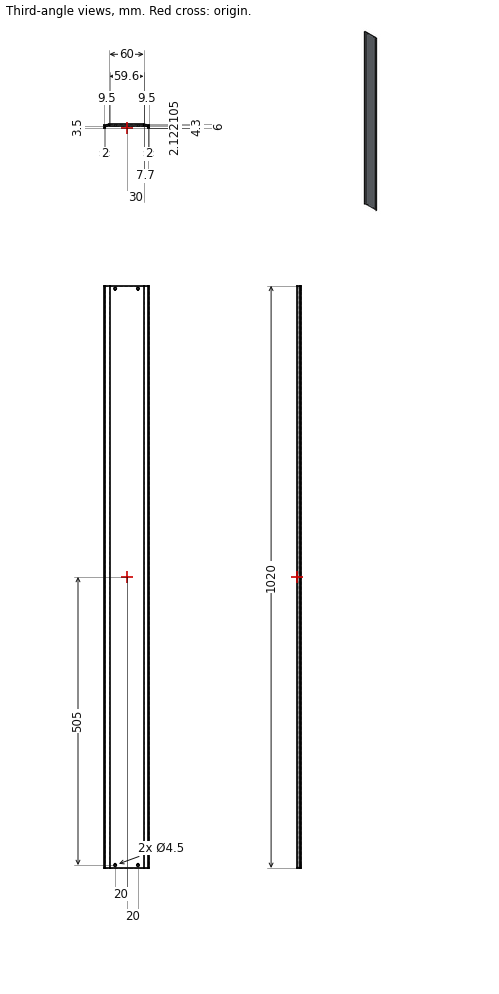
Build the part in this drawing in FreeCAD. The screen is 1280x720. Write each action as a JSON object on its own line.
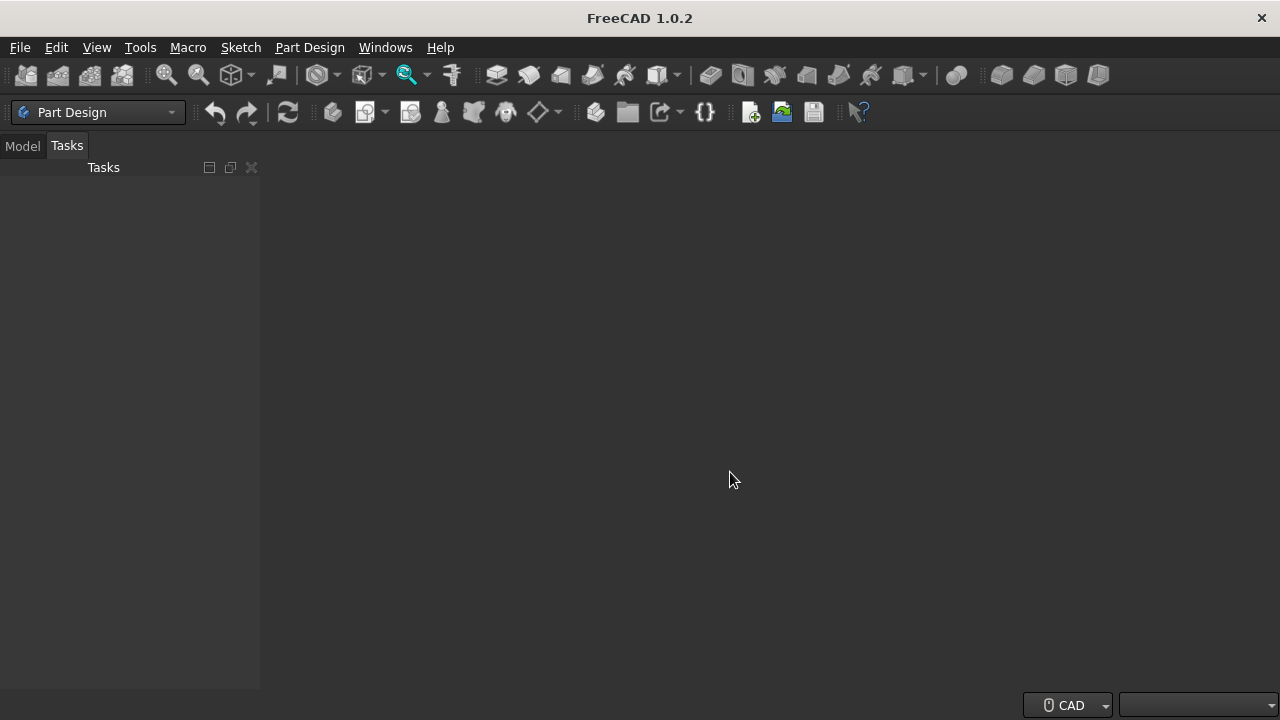
{"action": "key", "text": "ctrl+n"}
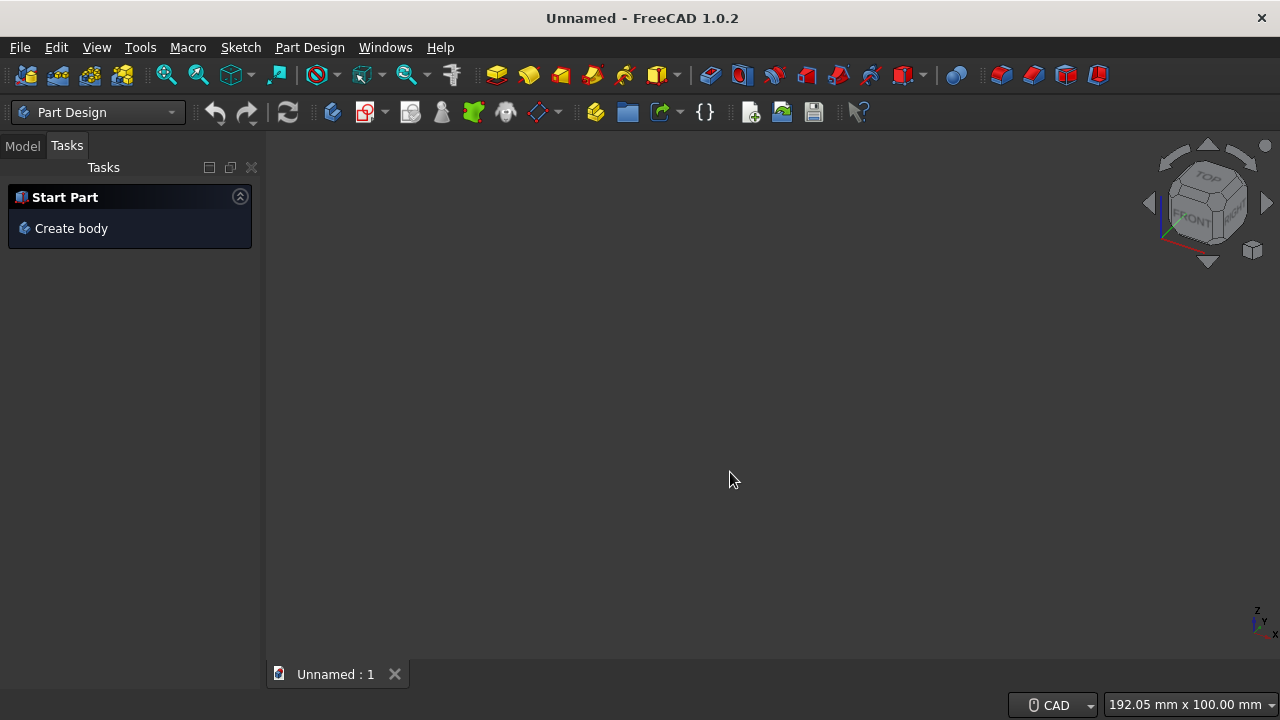
{"action": "left_click", "coordinate": [366, 112]}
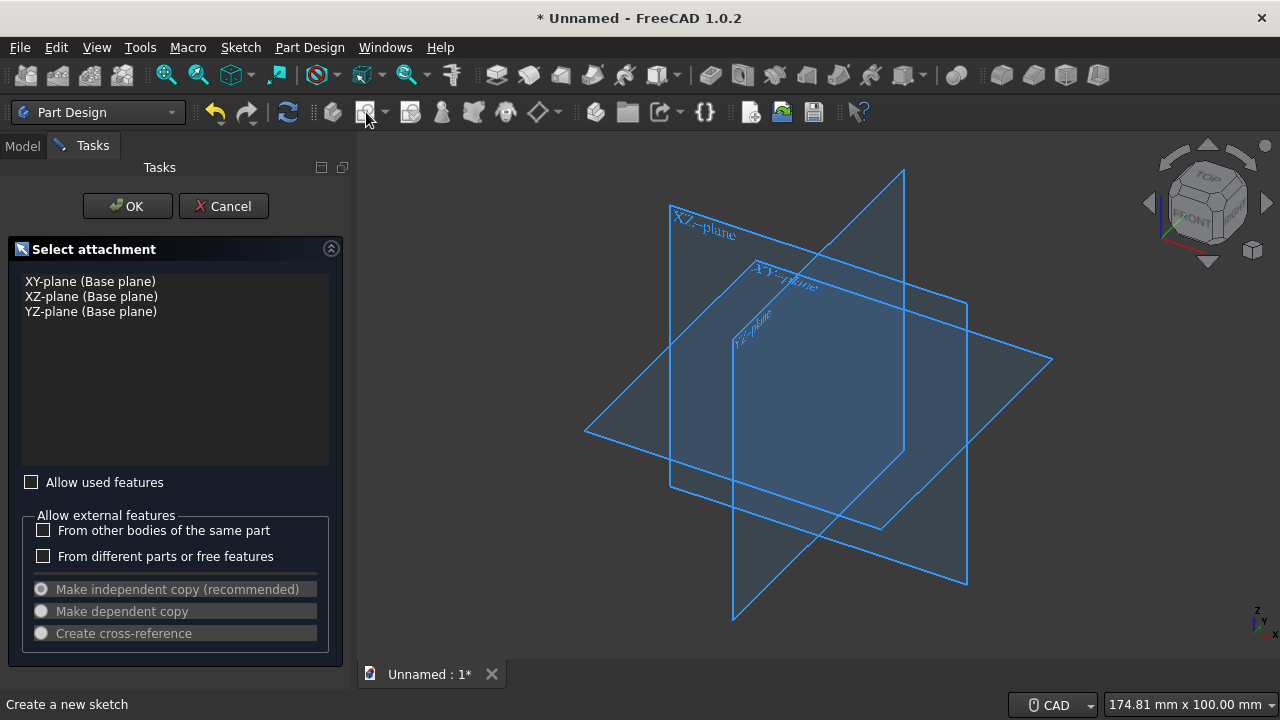
{"action": "left_click", "coordinate": [82, 282]}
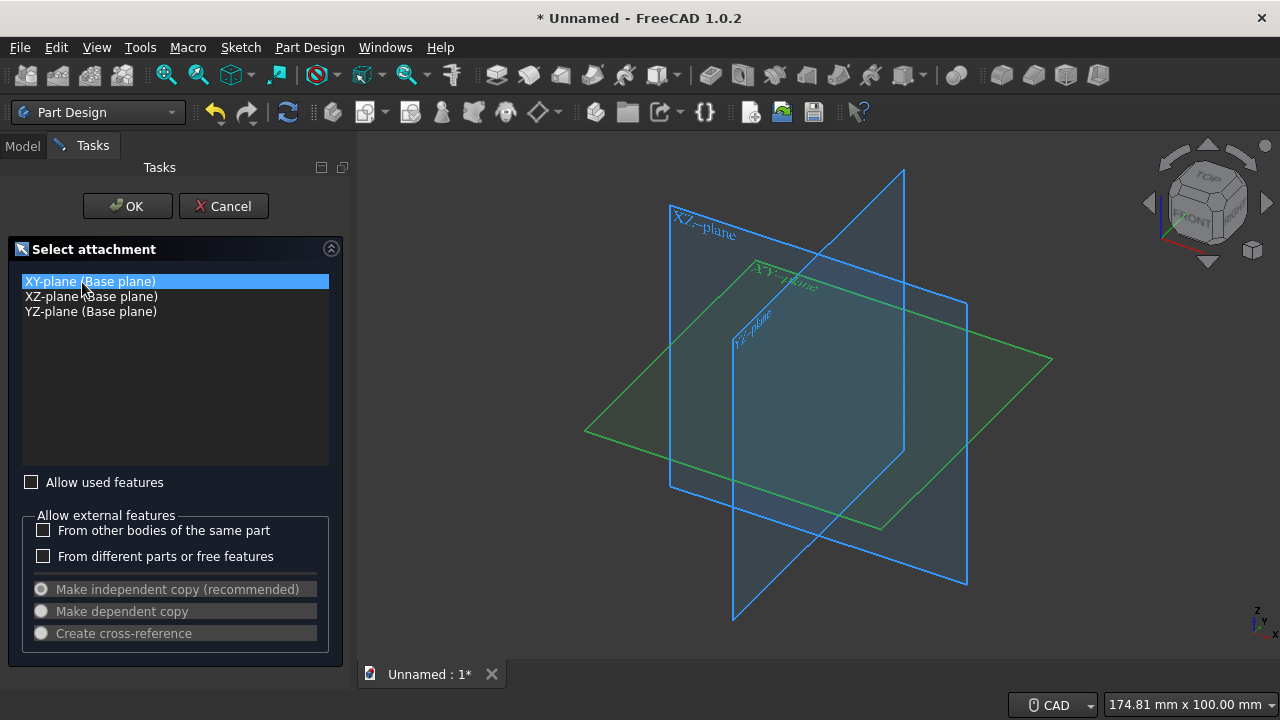
{"action": "left_click", "coordinate": [128, 206]}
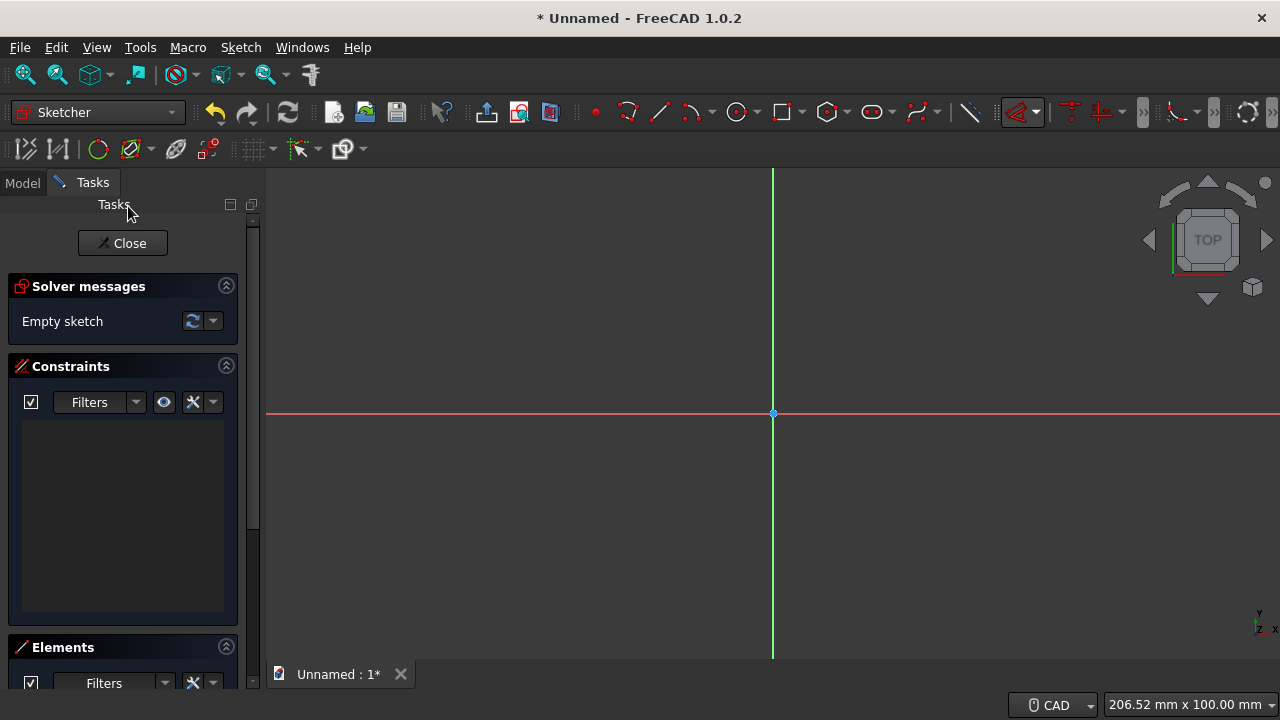
{"action": "scroll", "coordinate": [912, 369], "scroll_direction": "up", "scroll_amount": 2}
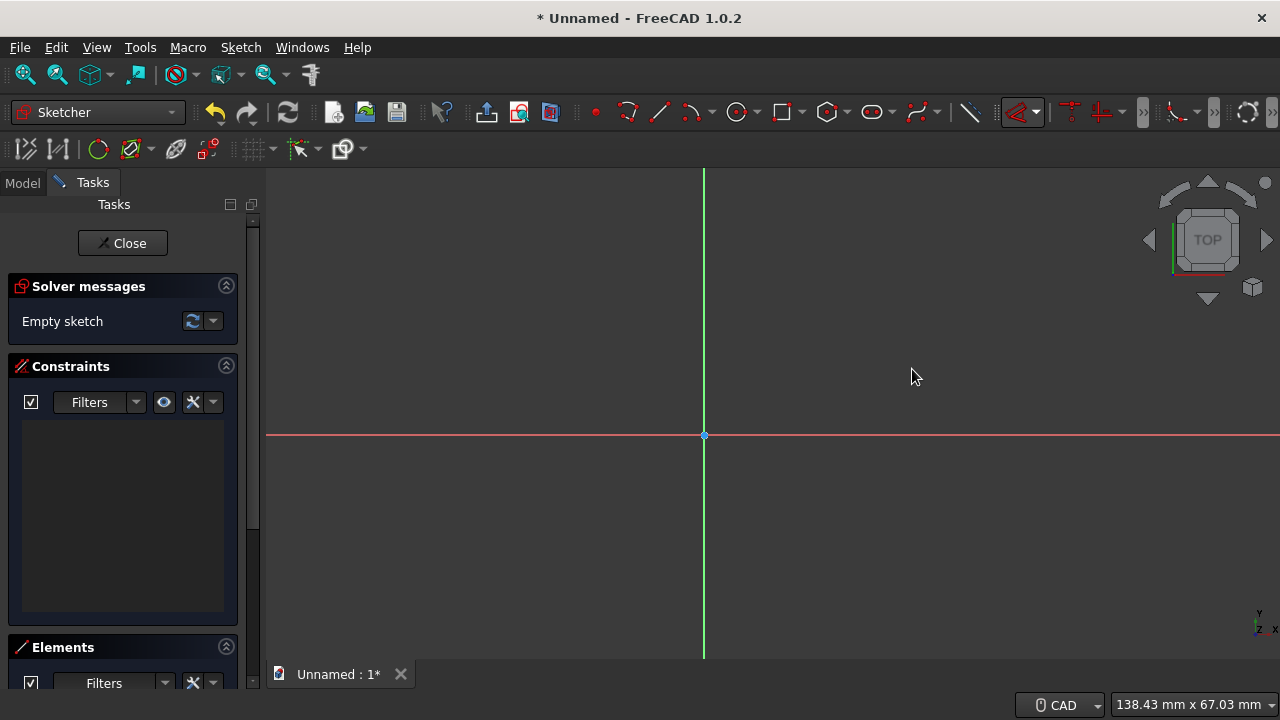
{"action": "key", "text": "g m"}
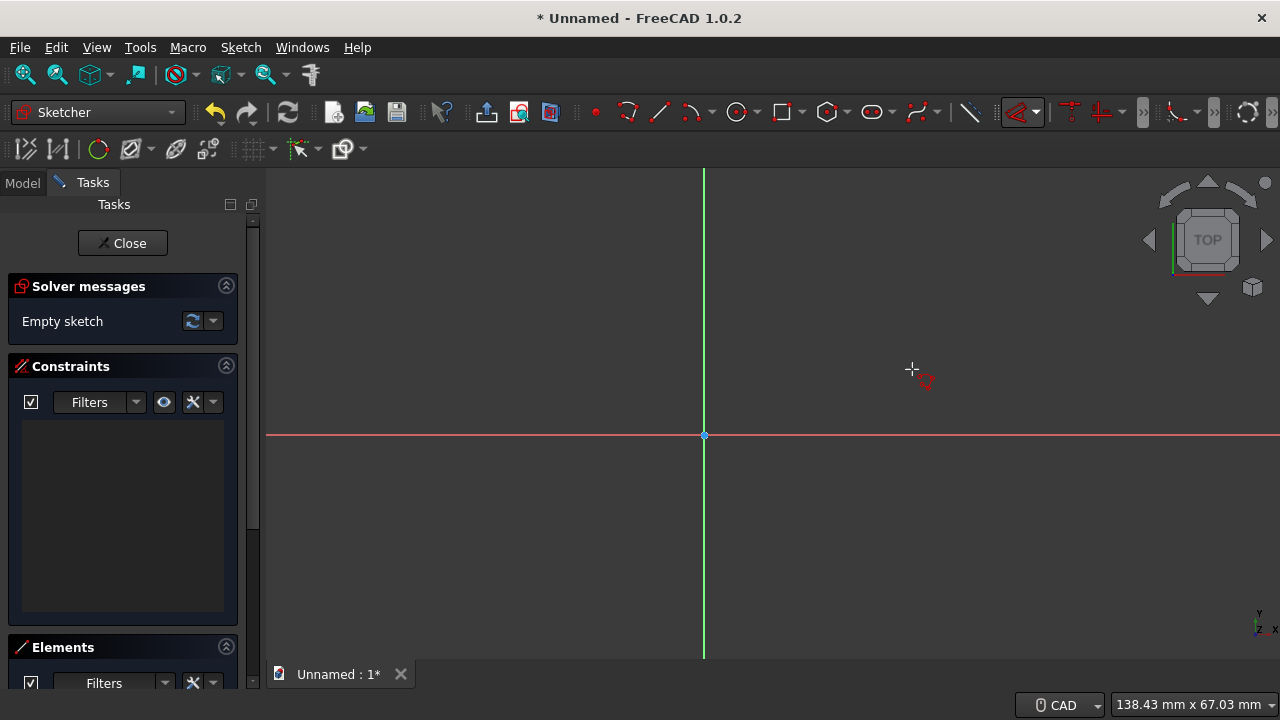
{"action": "left_click", "coordinate": [486, 410]}
{"action": "left_click", "coordinate": [923, 410]}
{"action": "left_click", "coordinate": [979, 420]}
{"action": "left_click", "coordinate": [979, 435]}
{"action": "left_click", "coordinate": [994, 426]}
{"action": "left_click", "coordinate": [994, 404]}
{"action": "left_click", "coordinate": [924, 391]}
{"action": "left_click", "coordinate": [485, 391]}
{"action": "left_click", "coordinate": [415, 404]}
{"action": "left_click", "coordinate": [415, 435]}
{"action": "left_click", "coordinate": [430, 426]}
{"action": "left_click", "coordinate": [430, 420]}
{"action": "left_click", "coordinate": [486, 411]}
{"action": "key", "text": "Escape"}
{"action": "key", "text": "Escape"}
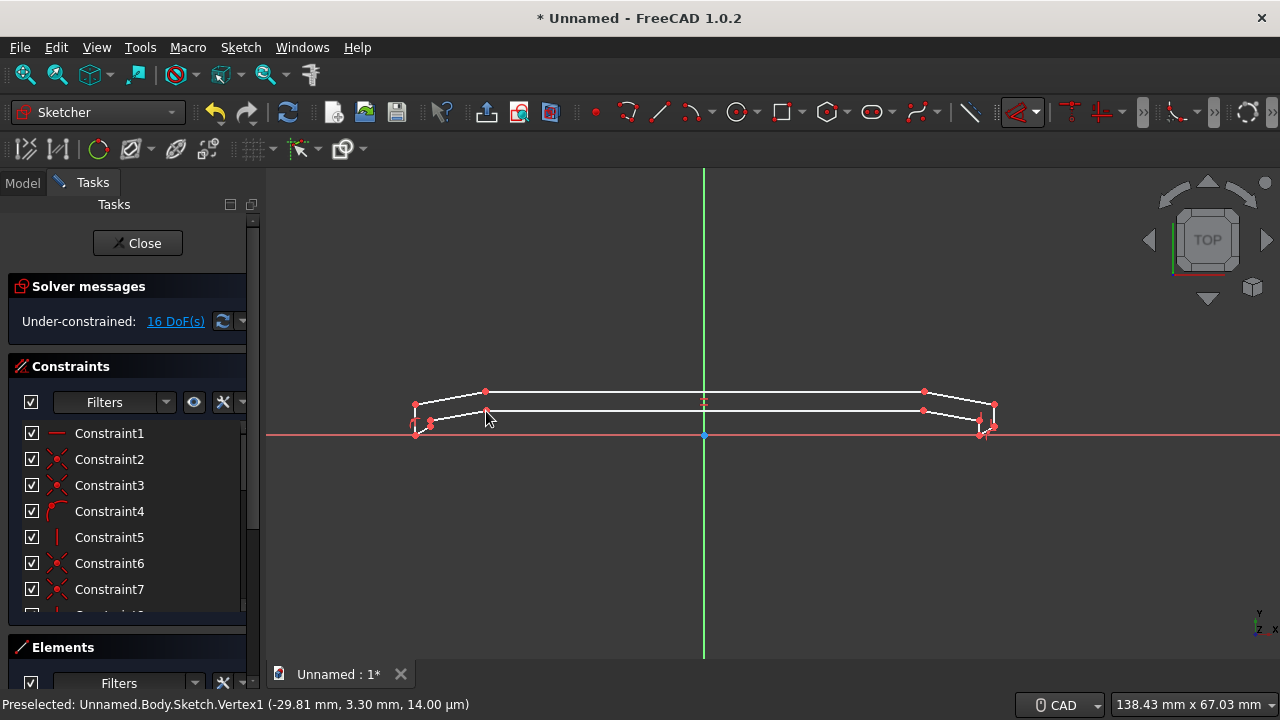
{"action": "scroll", "coordinate": [985, 432], "scroll_direction": "up", "scroll_amount": 5}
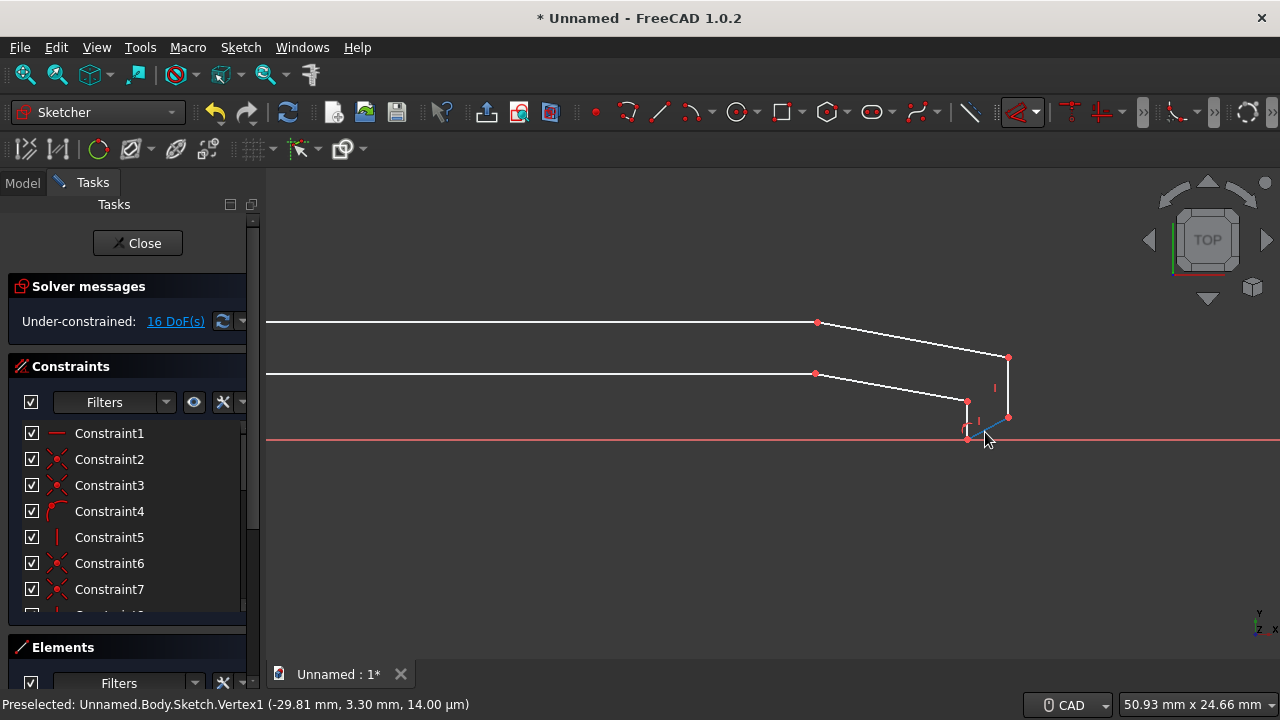
{"action": "left_click", "coordinate": [984, 431]}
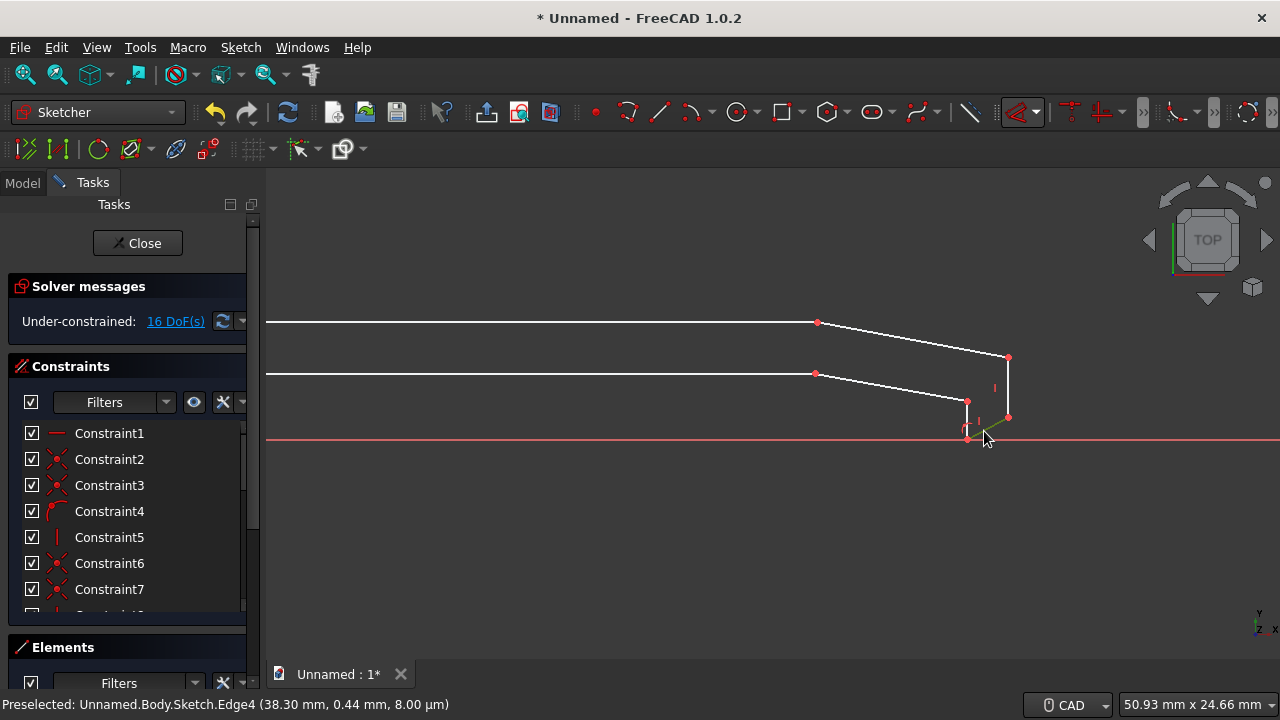
{"action": "key", "text": "h"}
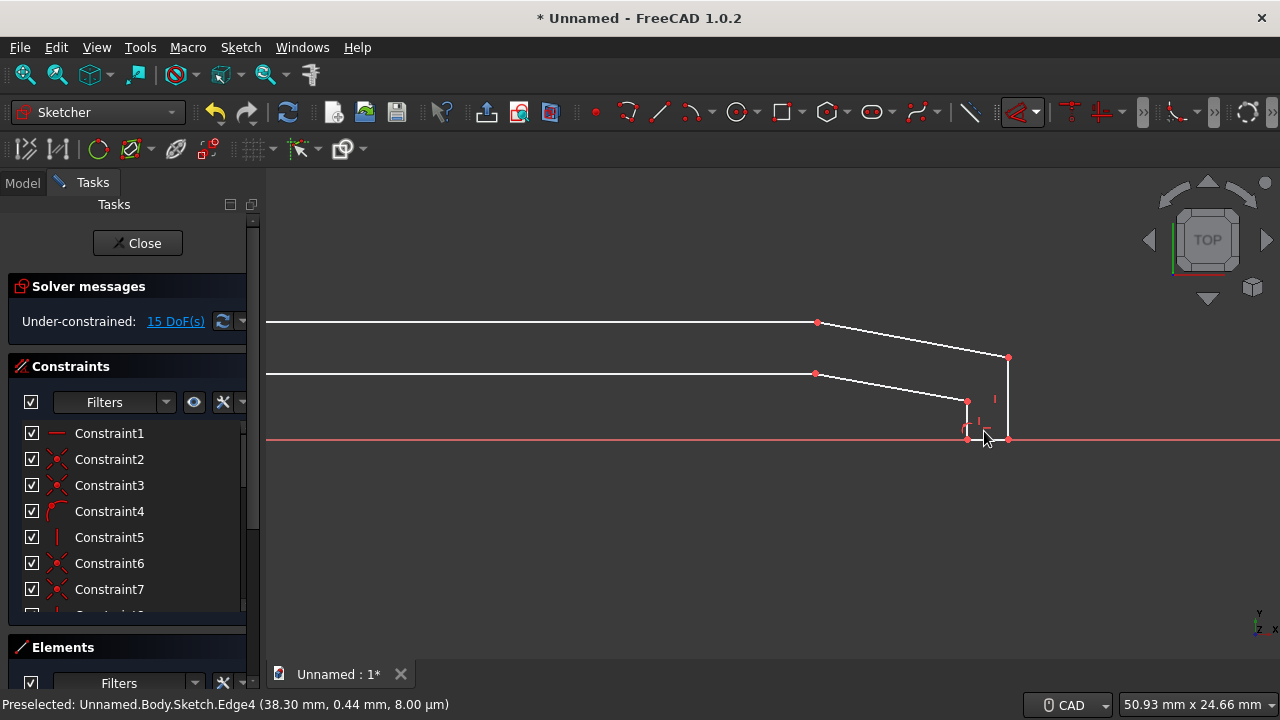
{"action": "scroll", "coordinate": [986, 433], "scroll_direction": "down", "scroll_amount": 5}